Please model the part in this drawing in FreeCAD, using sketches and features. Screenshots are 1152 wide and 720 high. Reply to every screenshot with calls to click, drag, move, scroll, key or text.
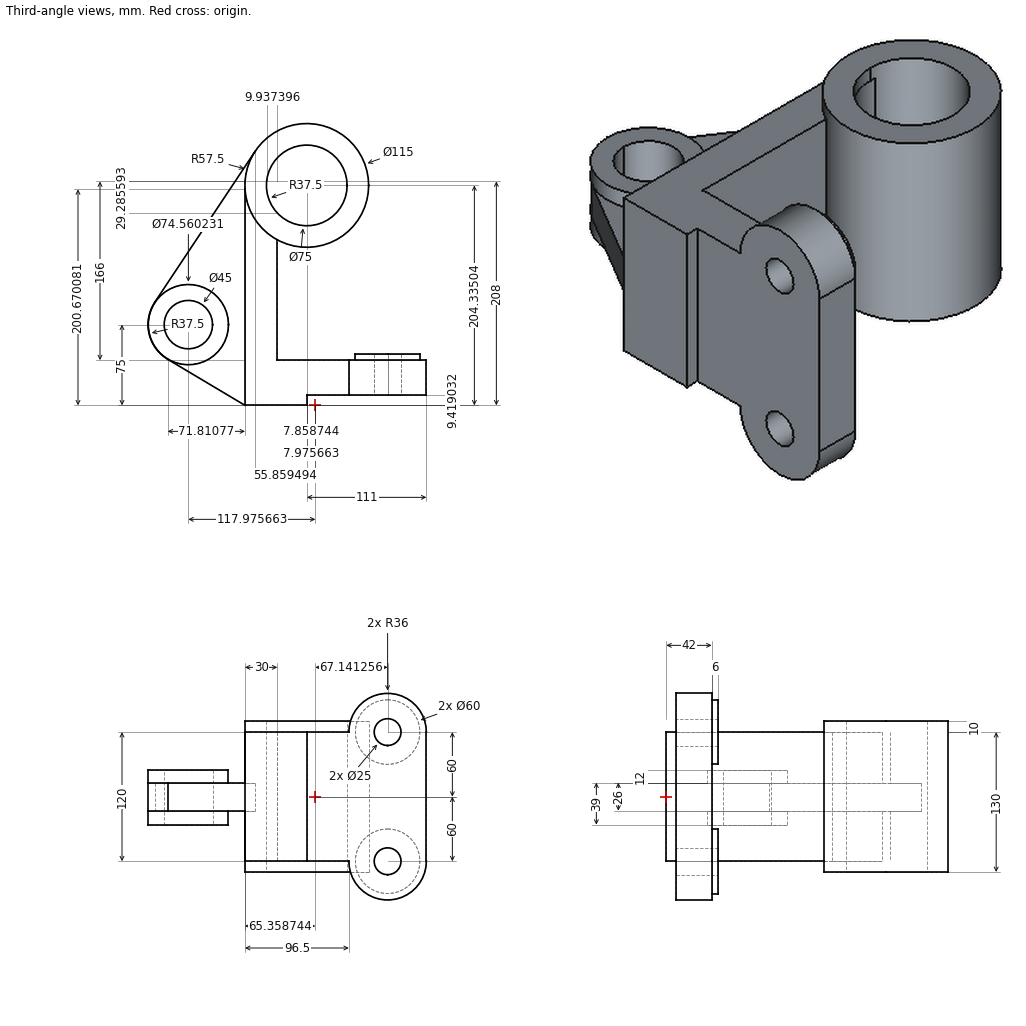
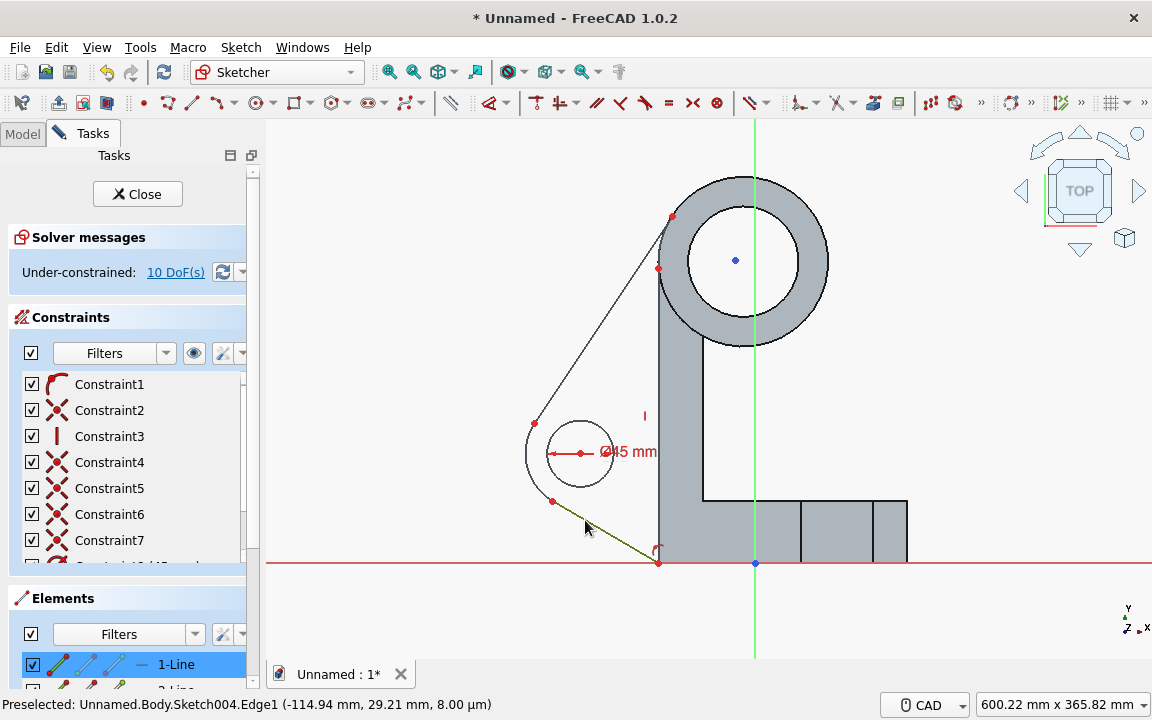
click(526, 448)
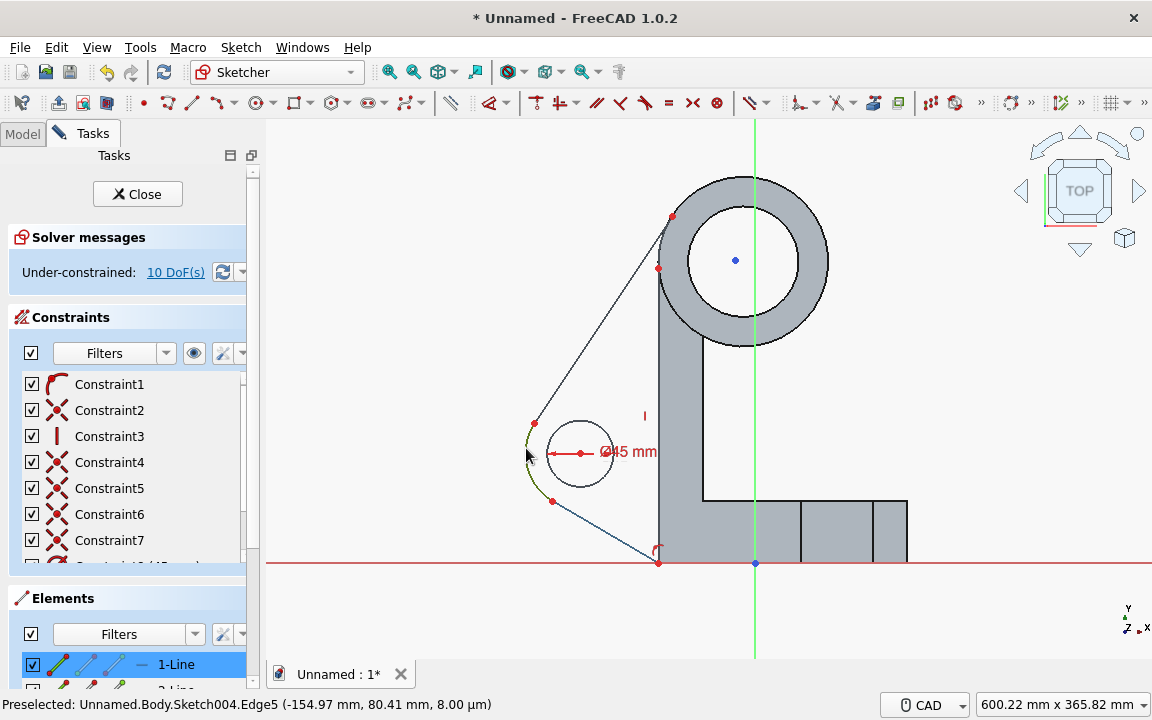
click(646, 104)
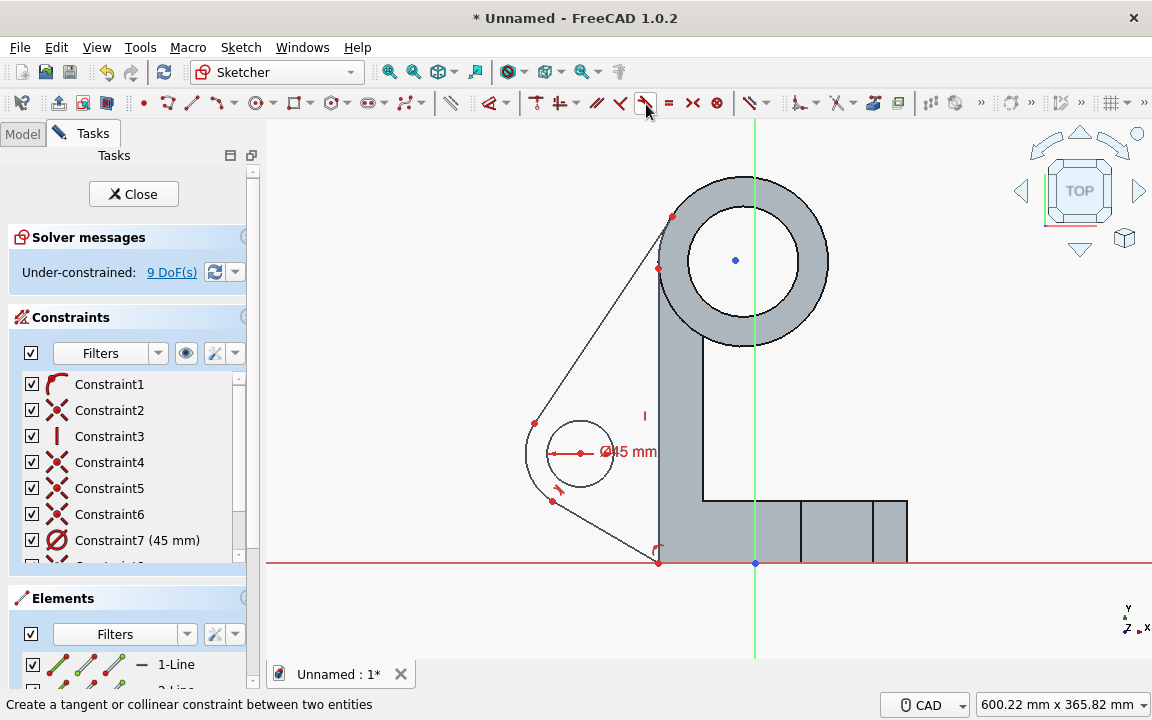
click(632, 278)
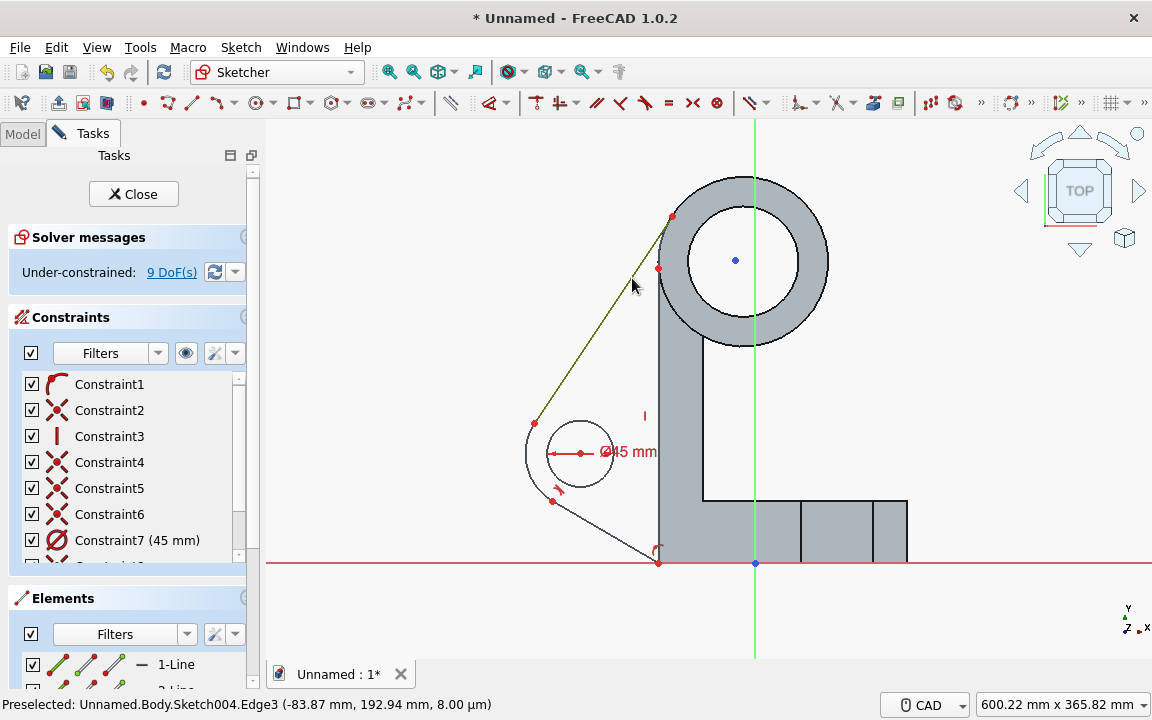
click(526, 448)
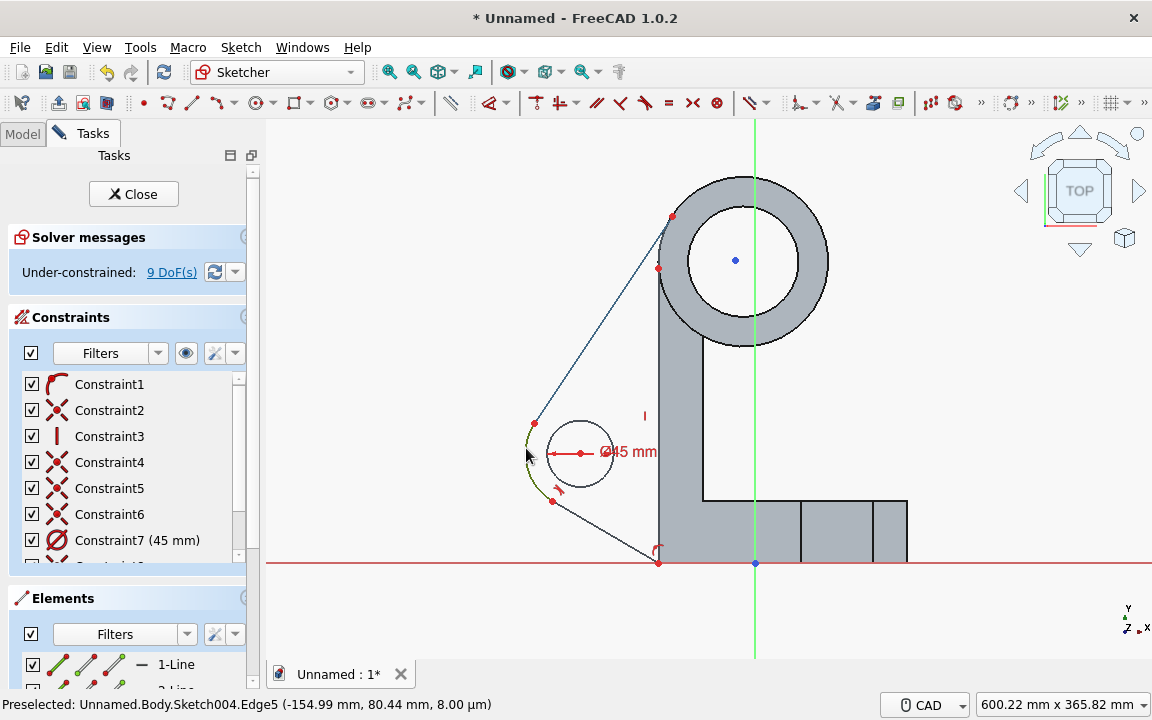
click(646, 104)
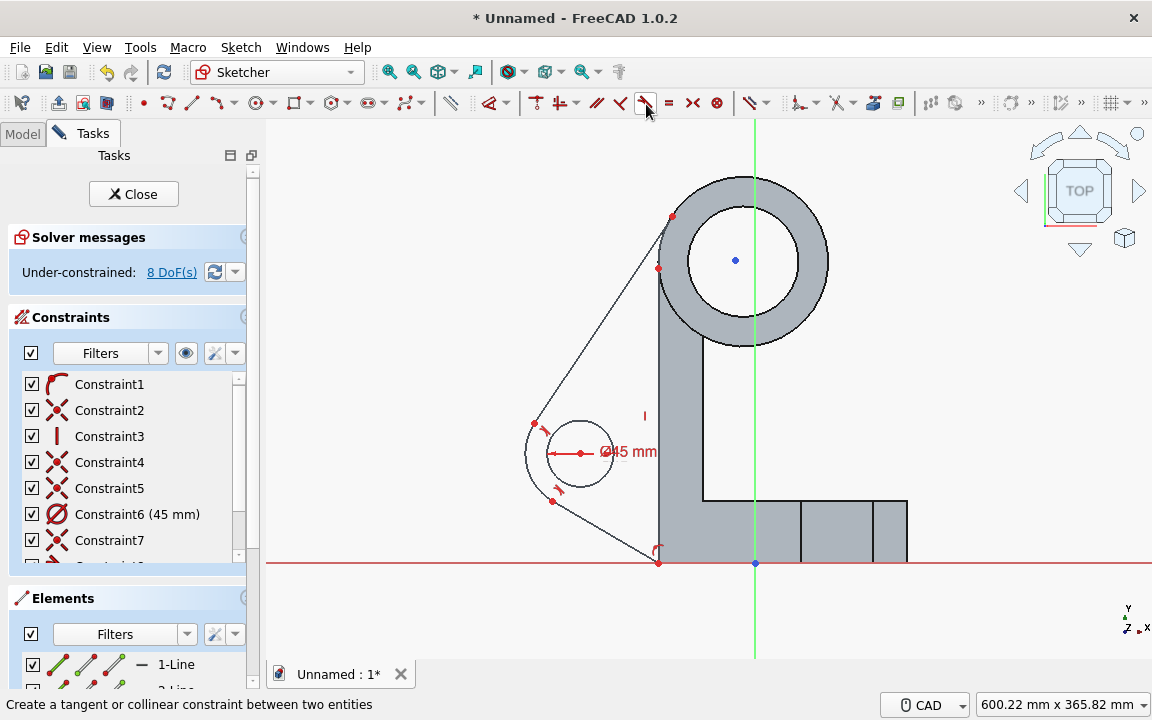
click(490, 104)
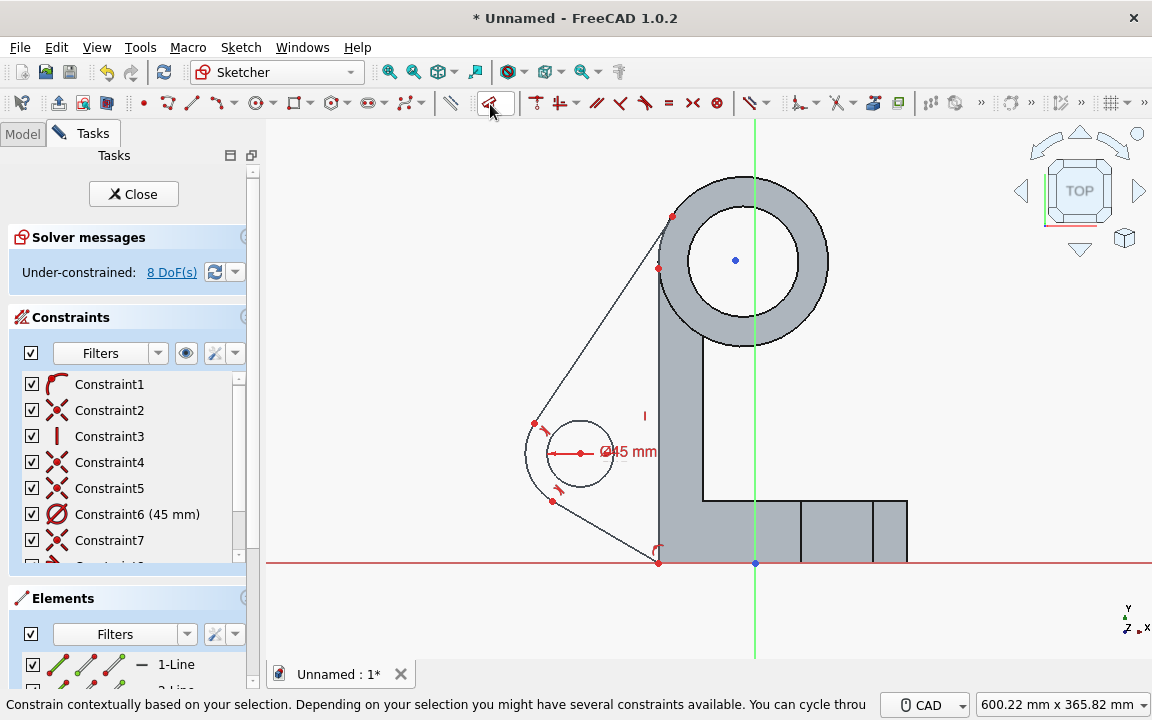
scroll(659, 257, up, 2)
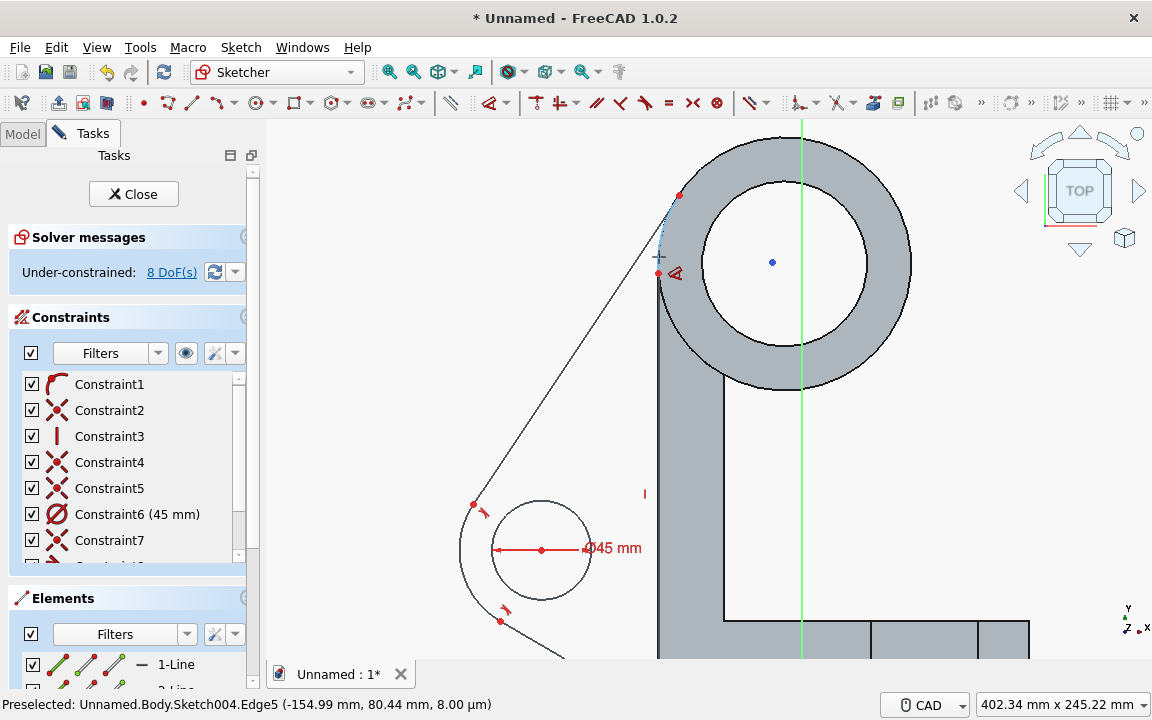
click(658, 257)
click(647, 186)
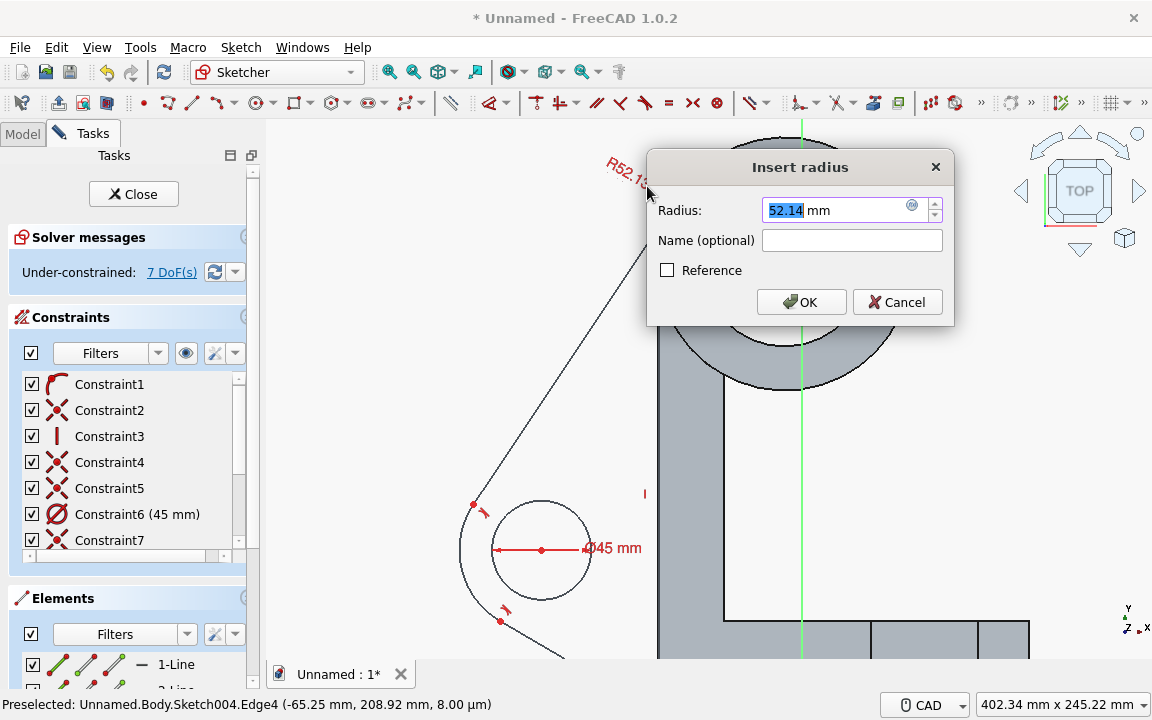
text(57.5)
key(Return)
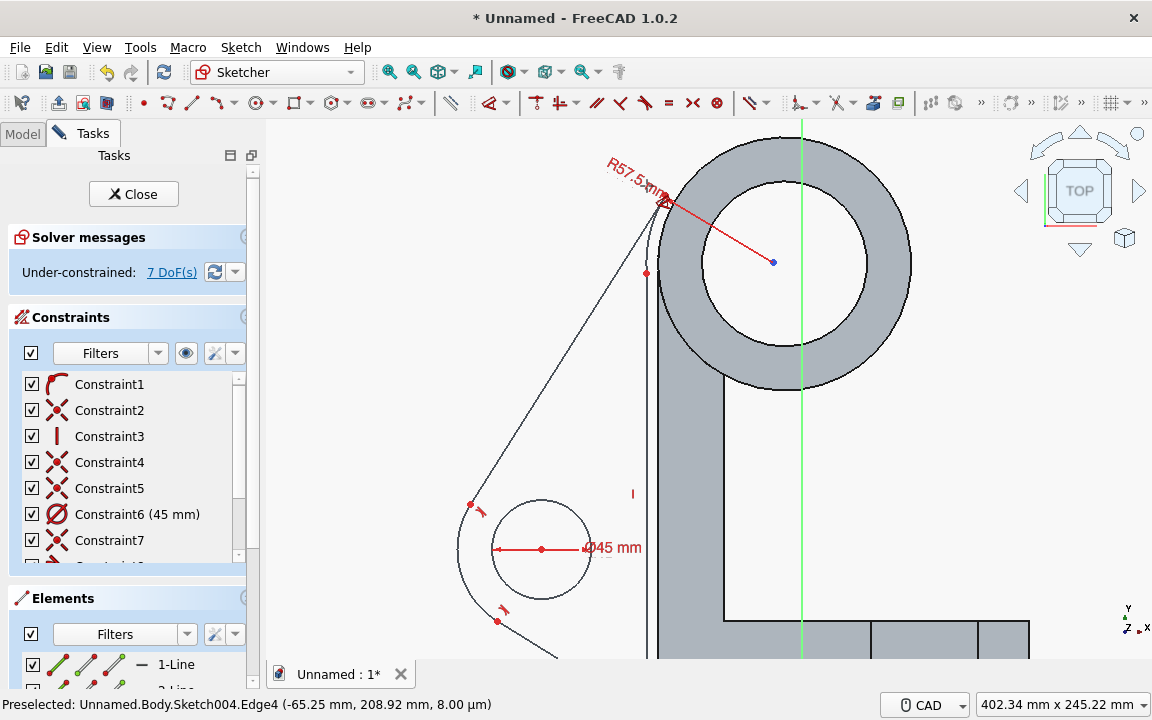
click(458, 542)
click(426, 539)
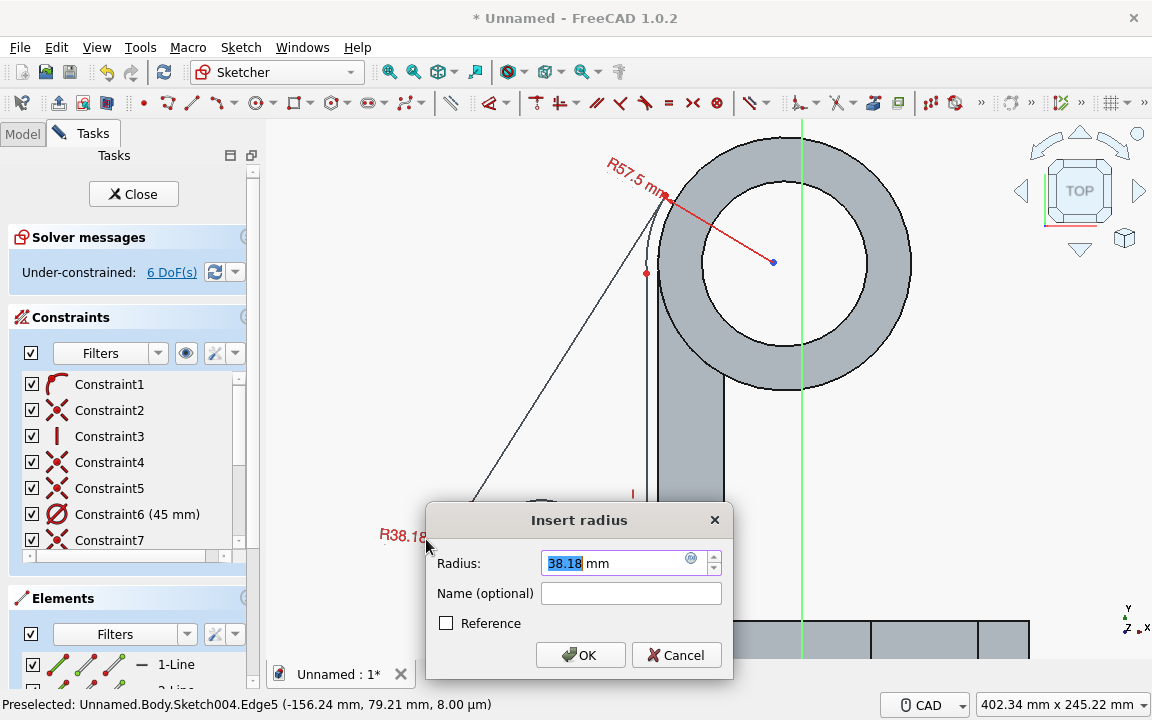
text(37.5)
key(Return)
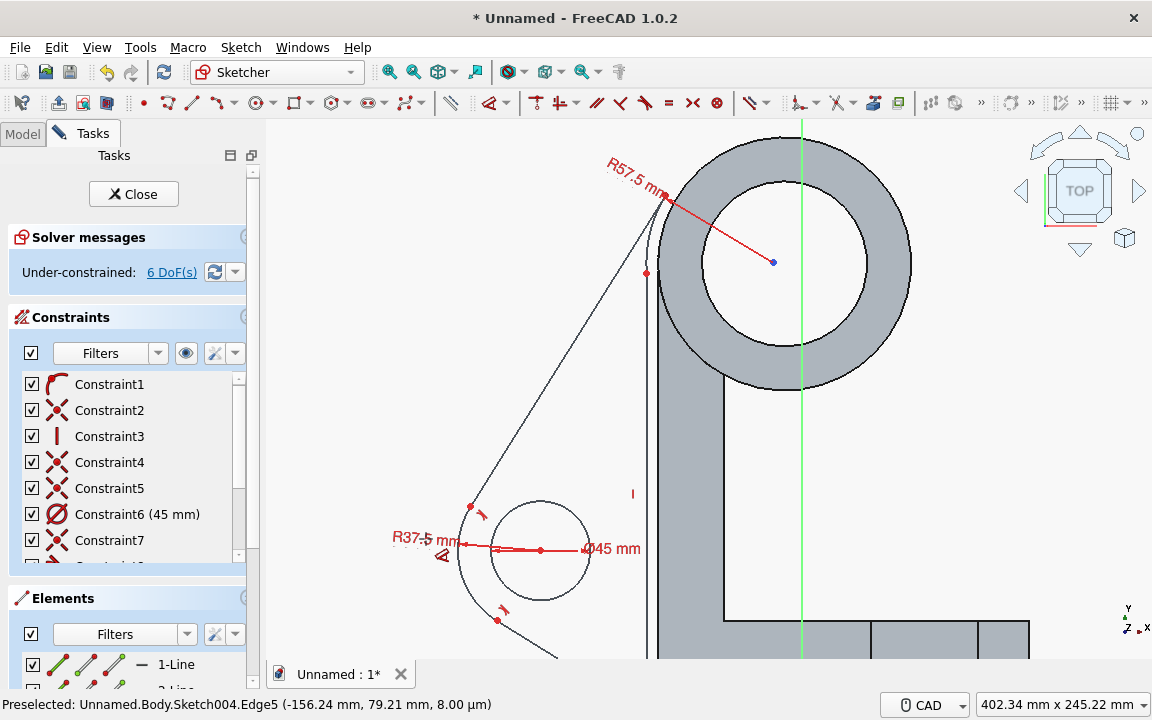
click(541, 551)
click(836, 591)